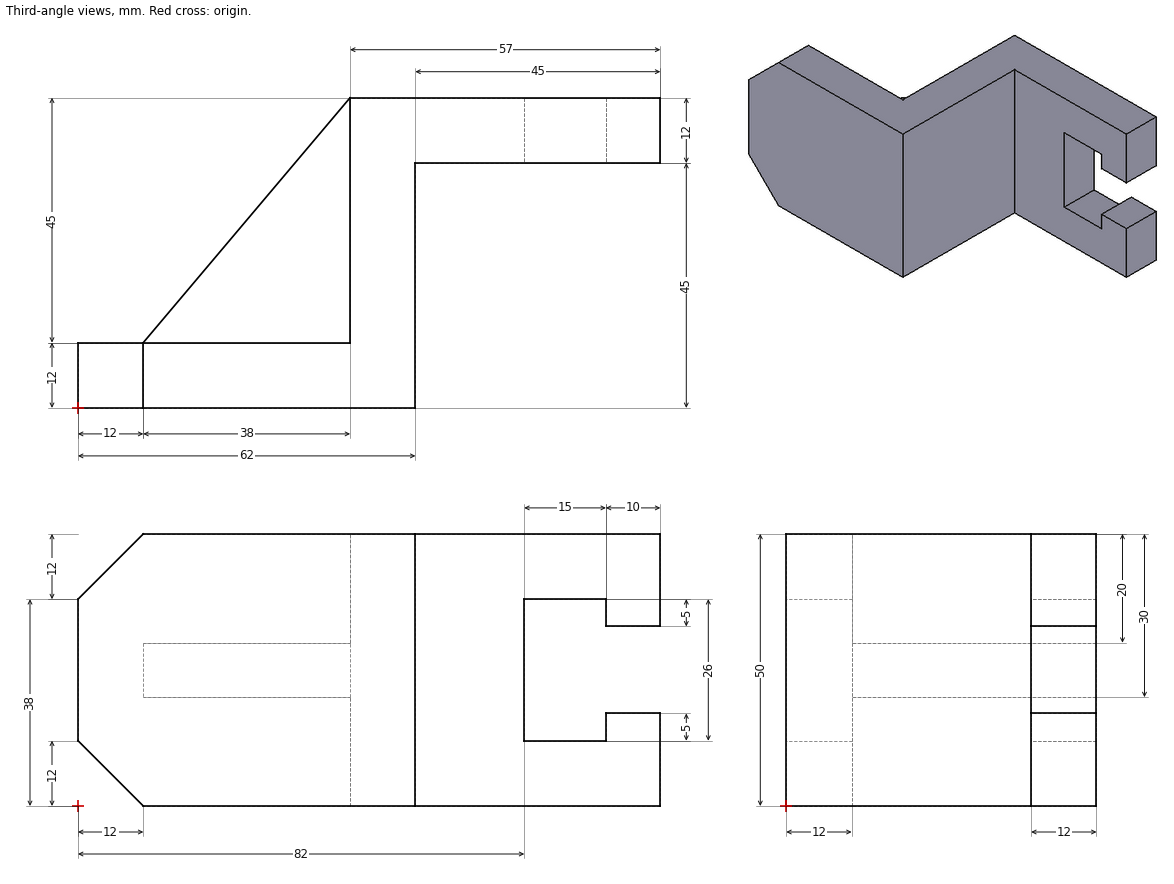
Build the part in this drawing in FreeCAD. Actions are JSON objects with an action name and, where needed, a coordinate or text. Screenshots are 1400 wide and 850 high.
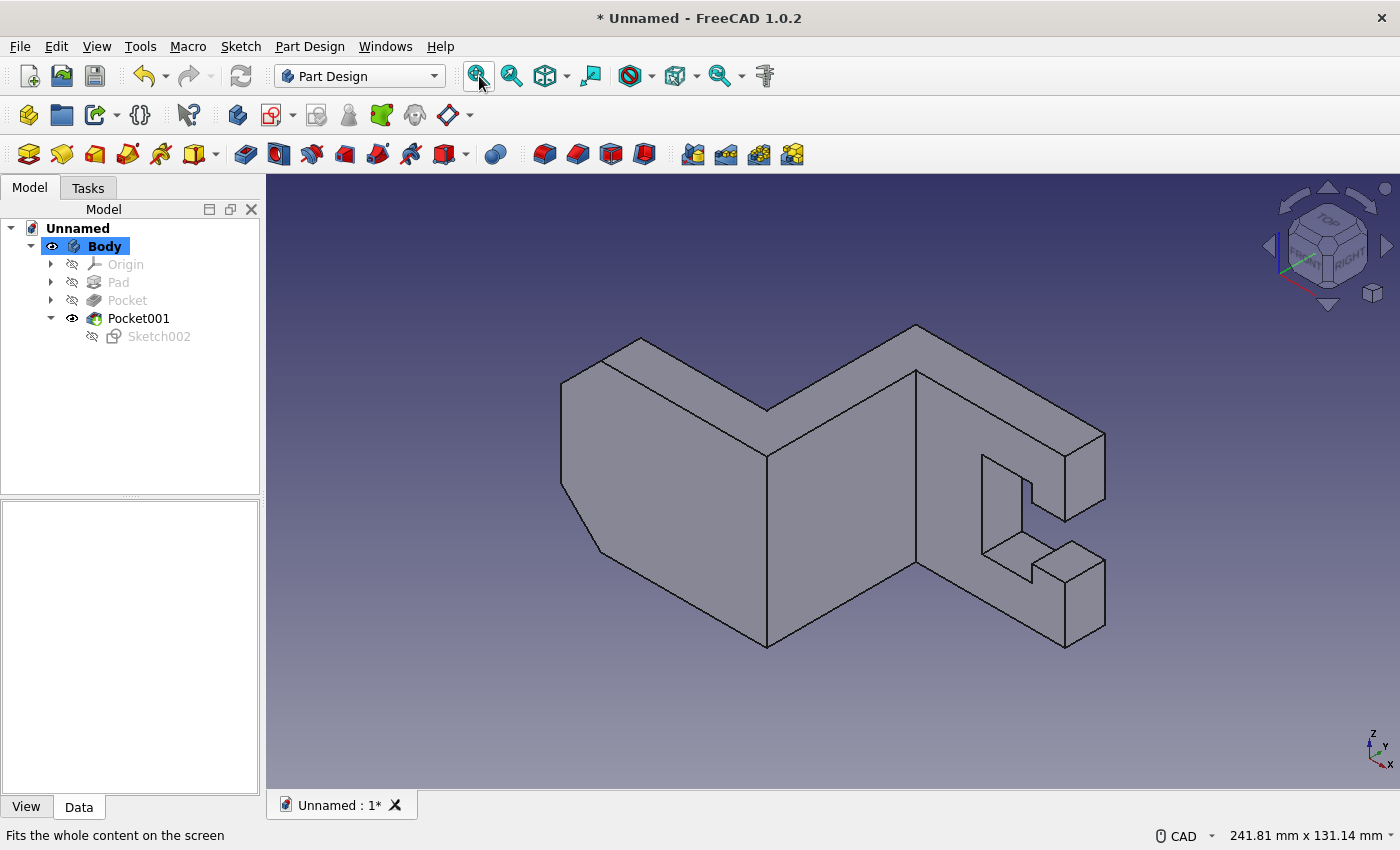
{"action": "left_click", "coordinate": [1069, 427]}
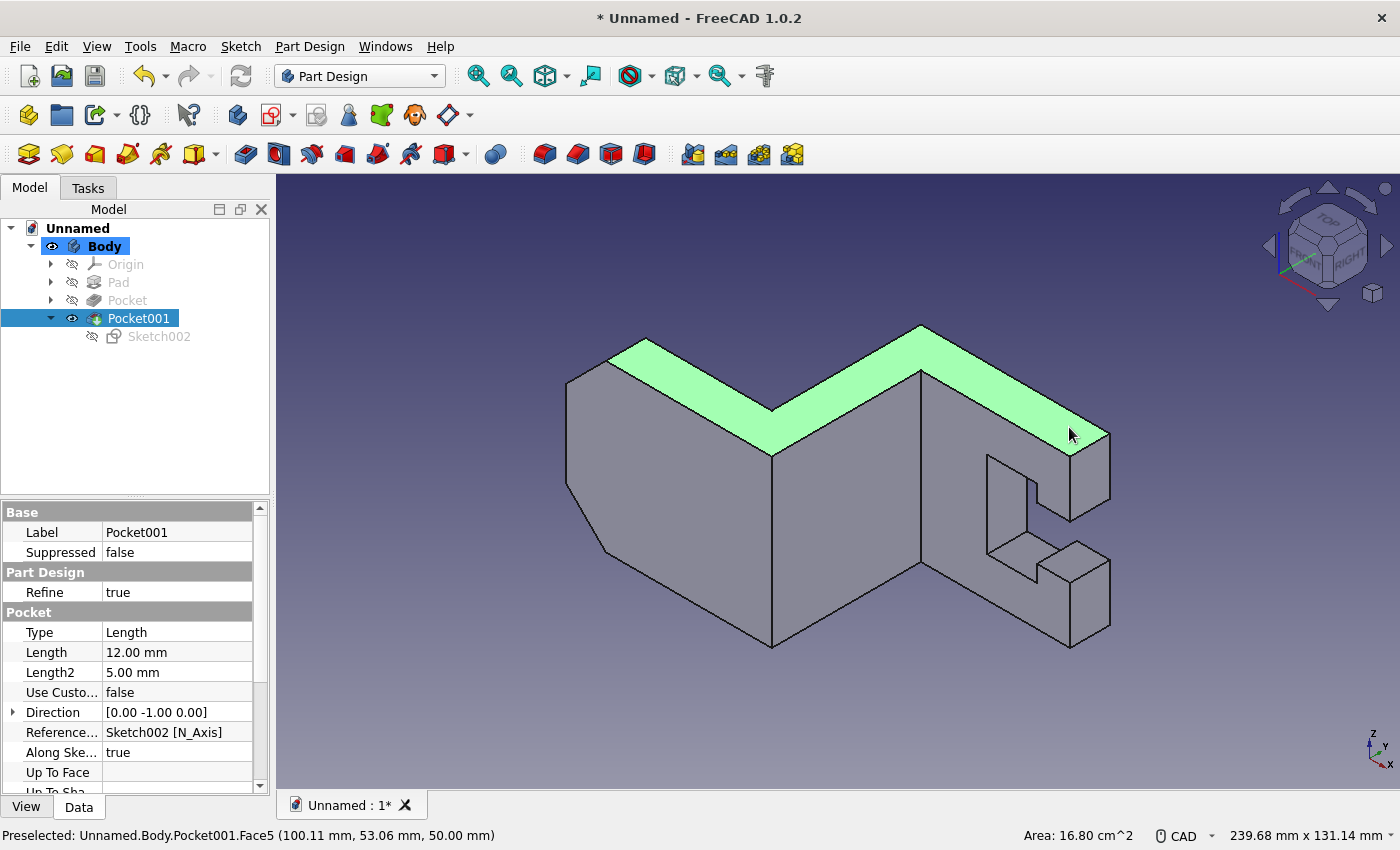
{"action": "left_click", "coordinate": [270, 116]}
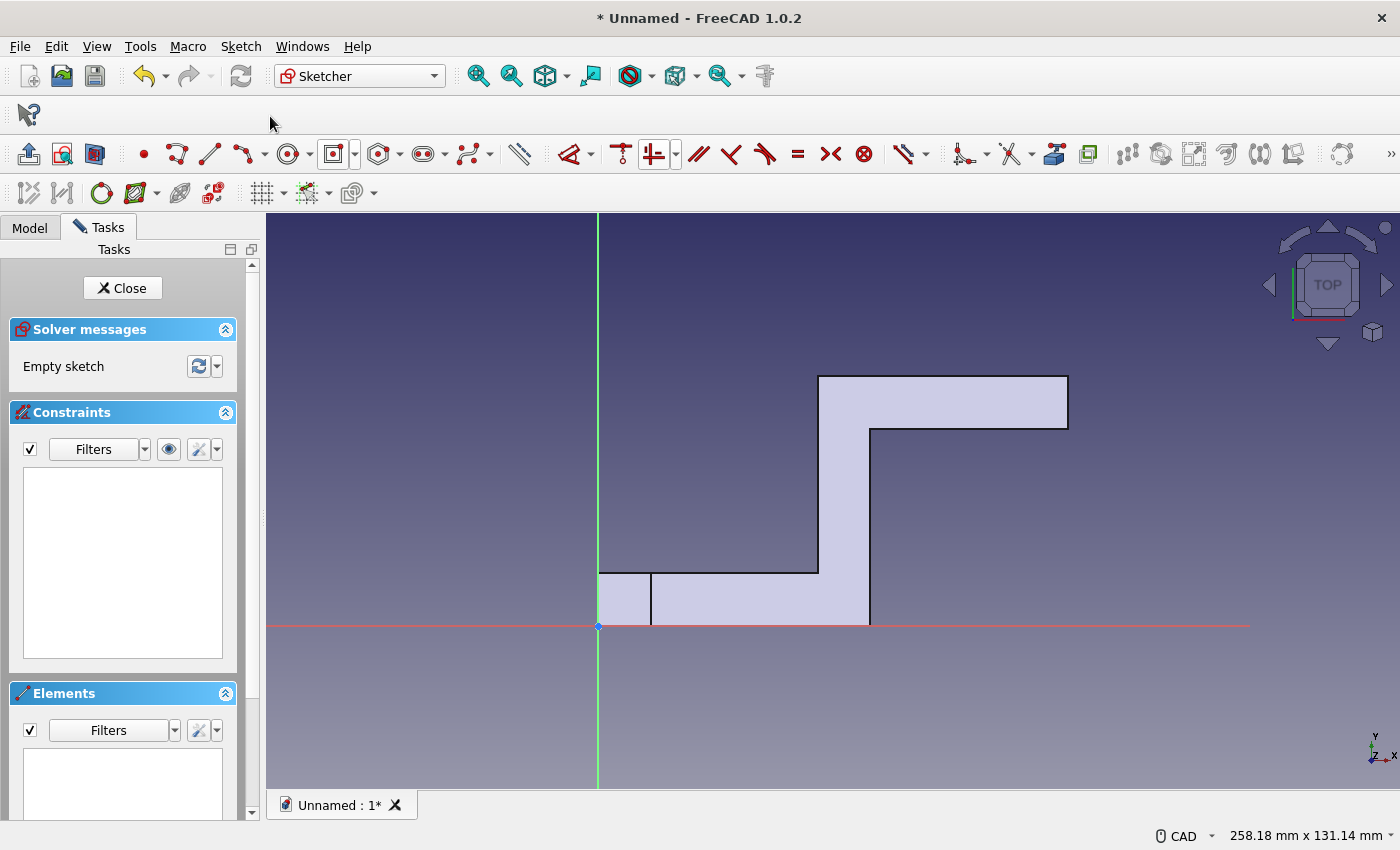
{"action": "scroll", "coordinate": [593, 501], "scroll_direction": "up", "scroll_amount": 2}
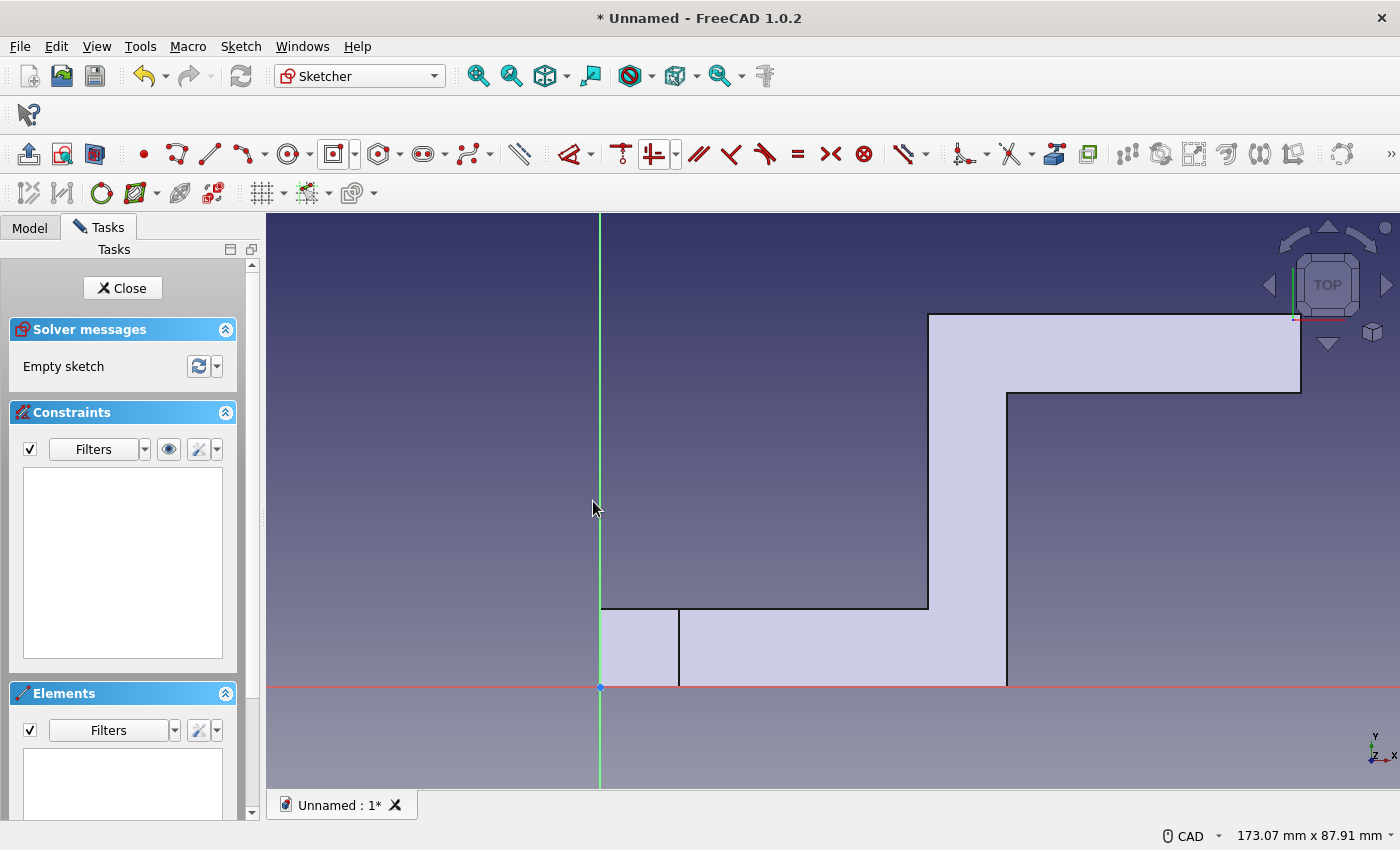
{"action": "left_click", "coordinate": [177, 154]}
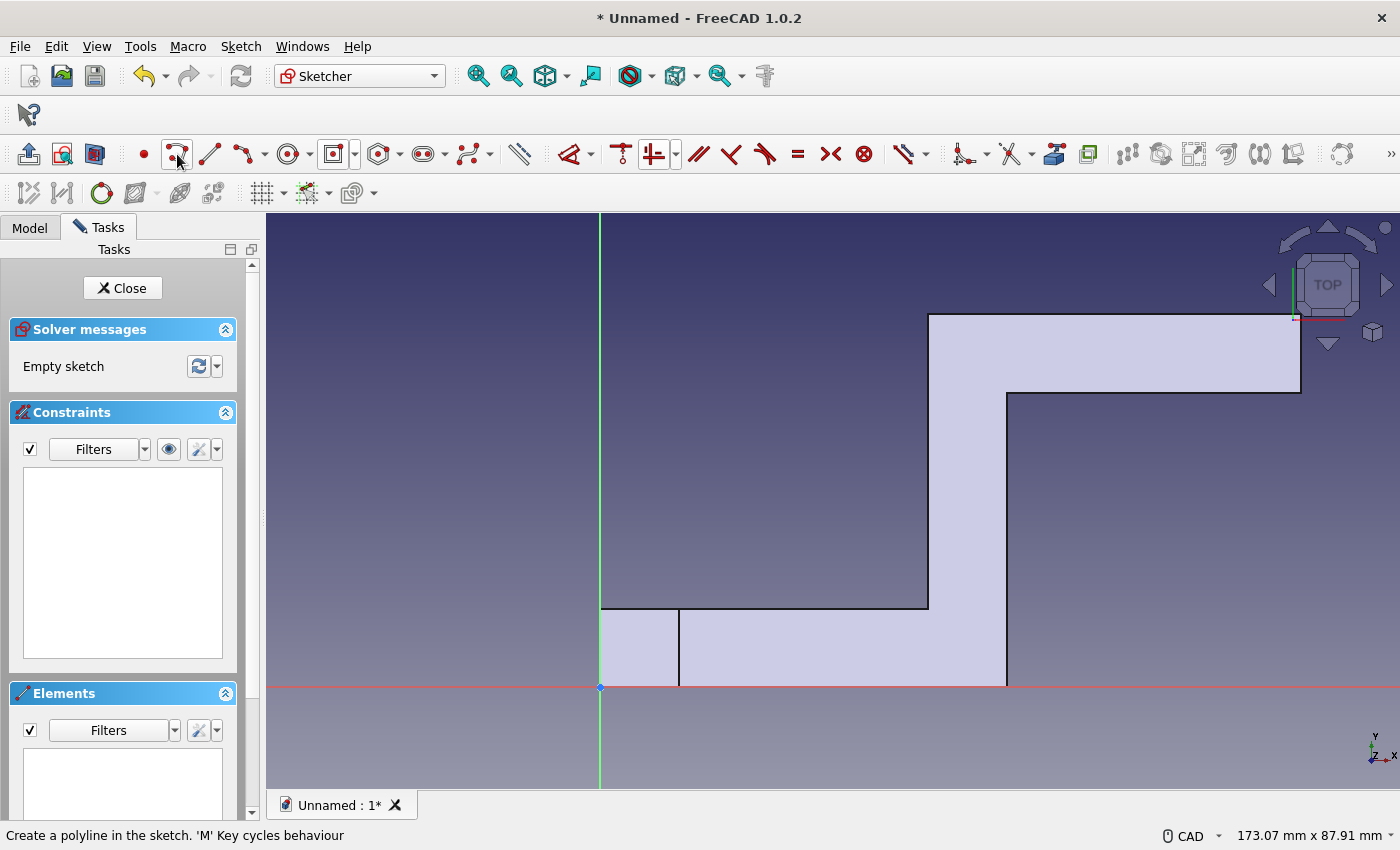
{"action": "left_click", "coordinate": [679, 609]}
{"action": "left_click", "coordinate": [928, 609]}
{"action": "left_click", "coordinate": [928, 314]}
{"action": "left_click", "coordinate": [679, 610]}
{"action": "key", "text": "Escape"}
{"action": "key", "text": "Escape"}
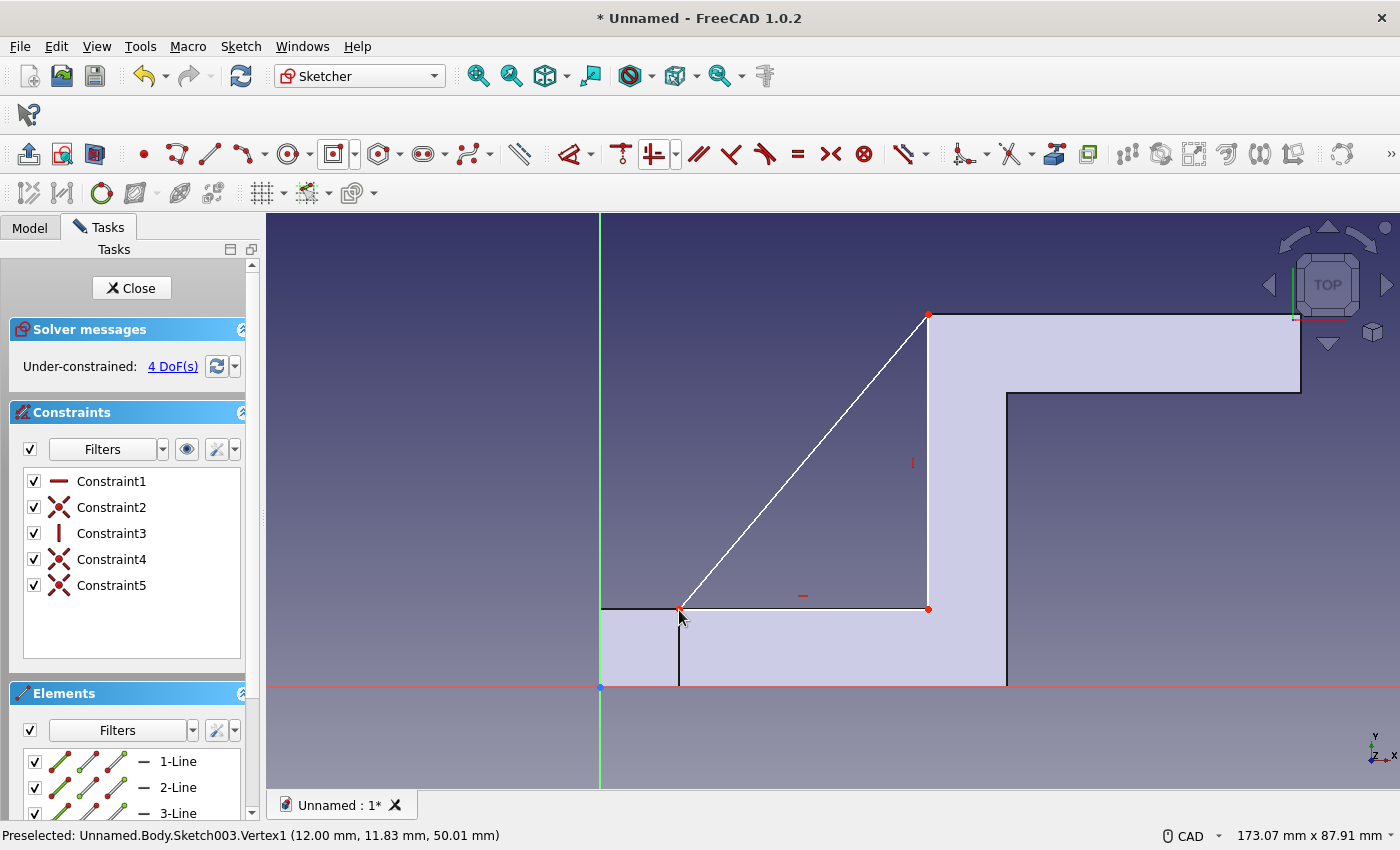
{"action": "left_click", "coordinate": [568, 154]}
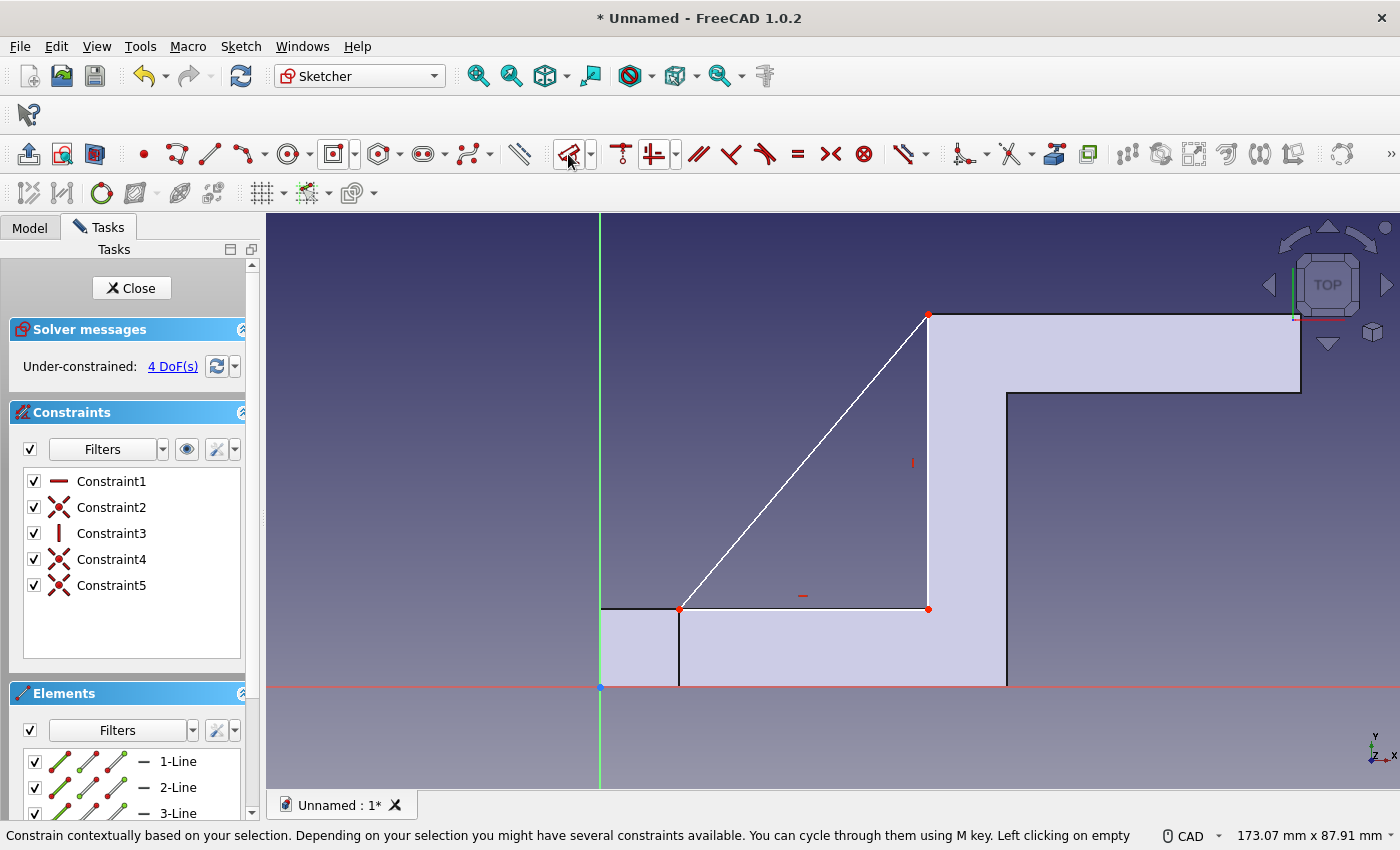
{"action": "left_click", "coordinate": [754, 610]}
{"action": "left_click", "coordinate": [804, 644]}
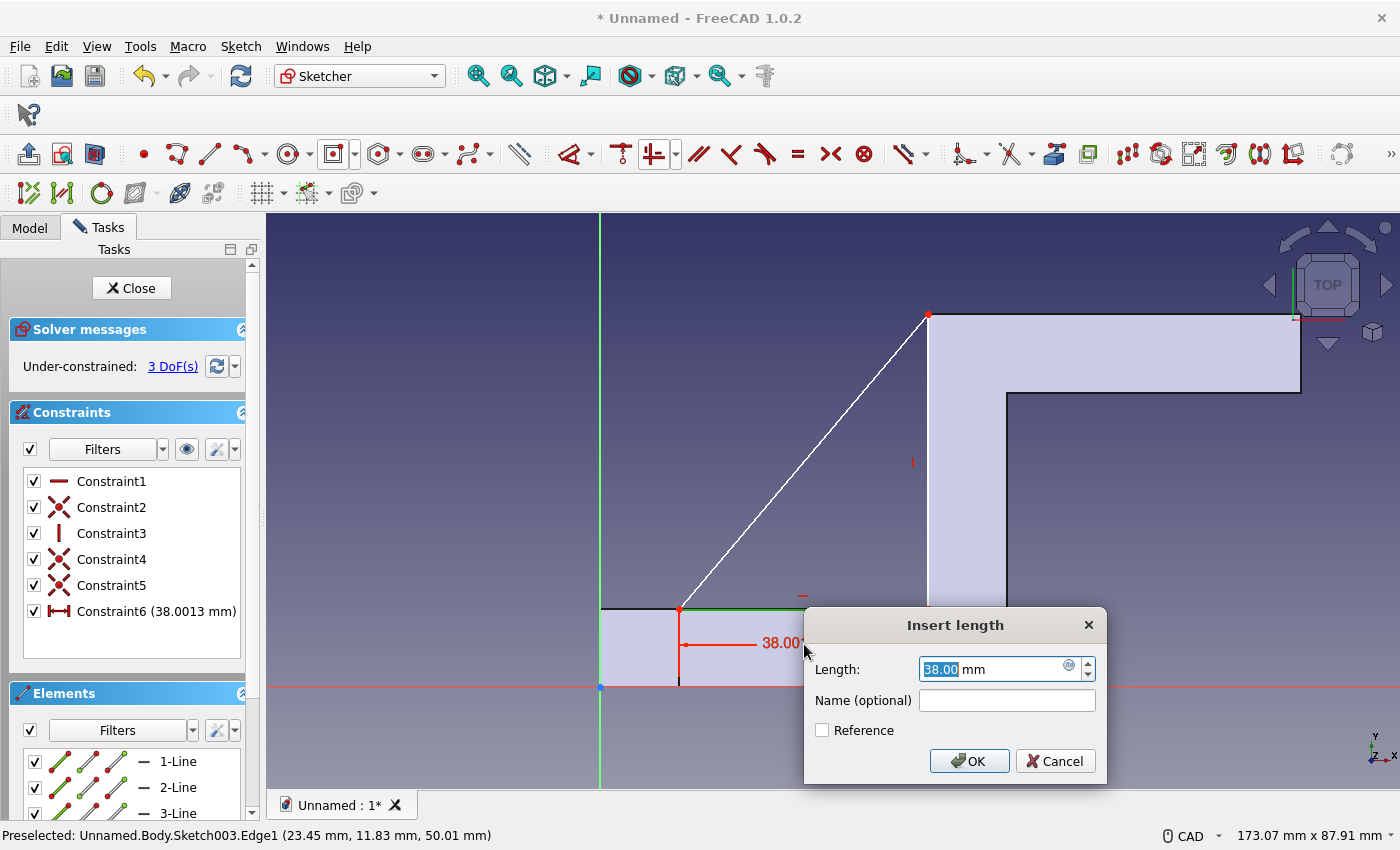
{"action": "type", "text": "38"}
{"action": "key", "text": "Return"}